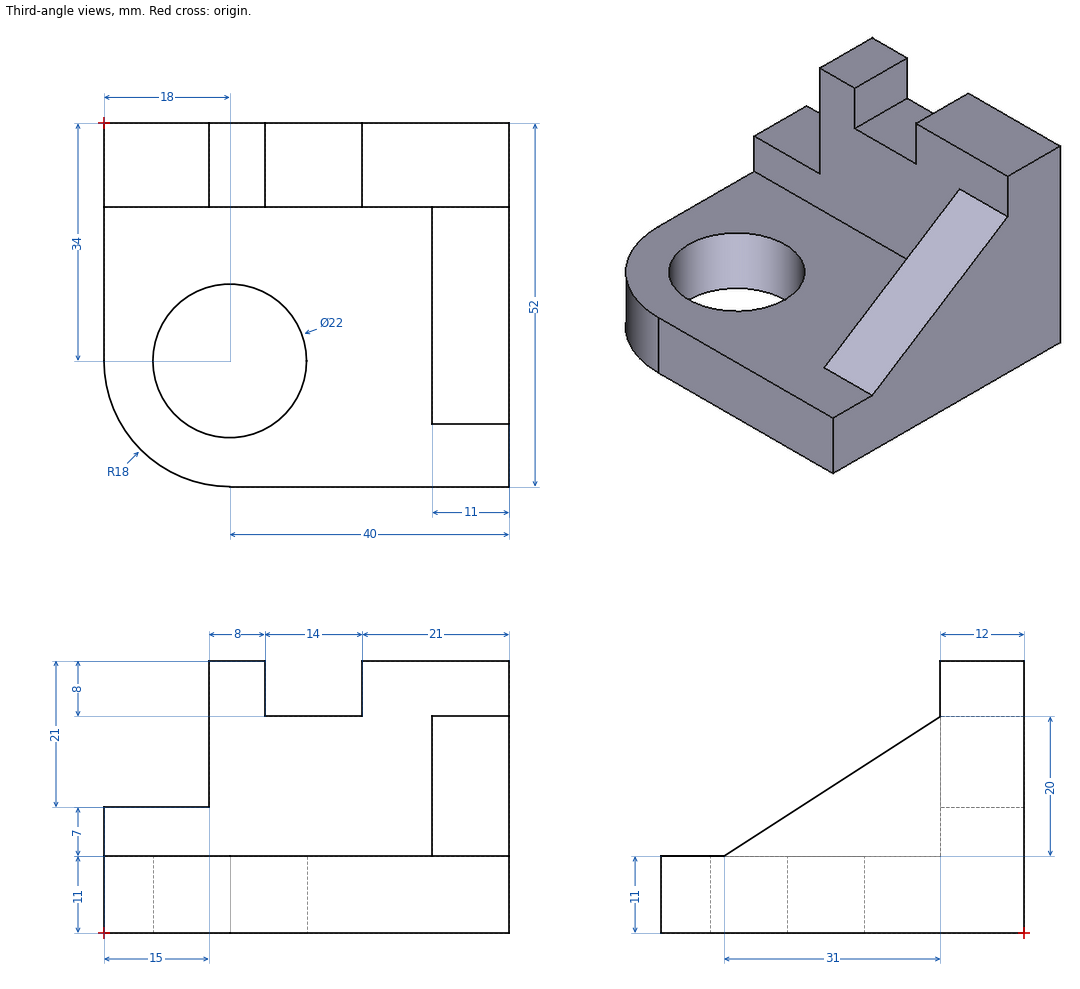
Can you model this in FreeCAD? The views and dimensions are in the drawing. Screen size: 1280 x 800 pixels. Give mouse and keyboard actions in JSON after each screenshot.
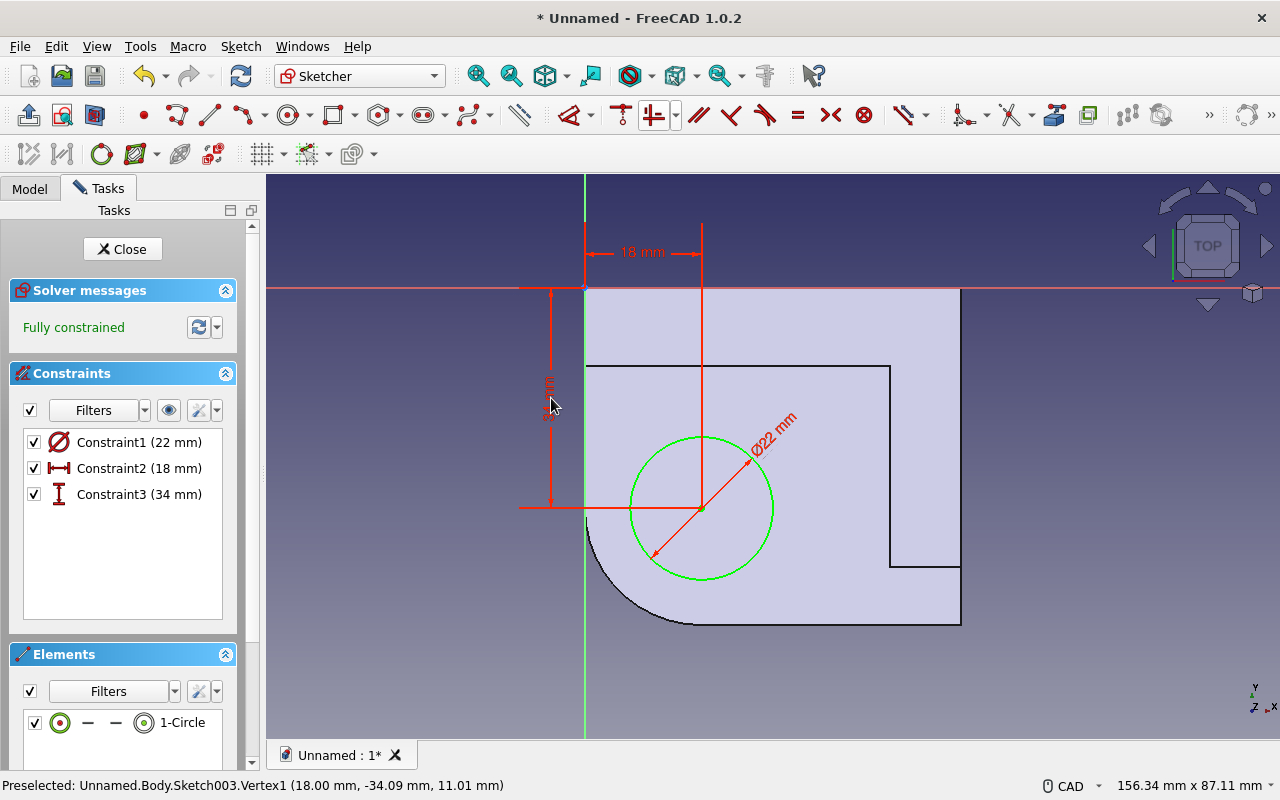
{"action": "left_click", "coordinate": [123, 249]}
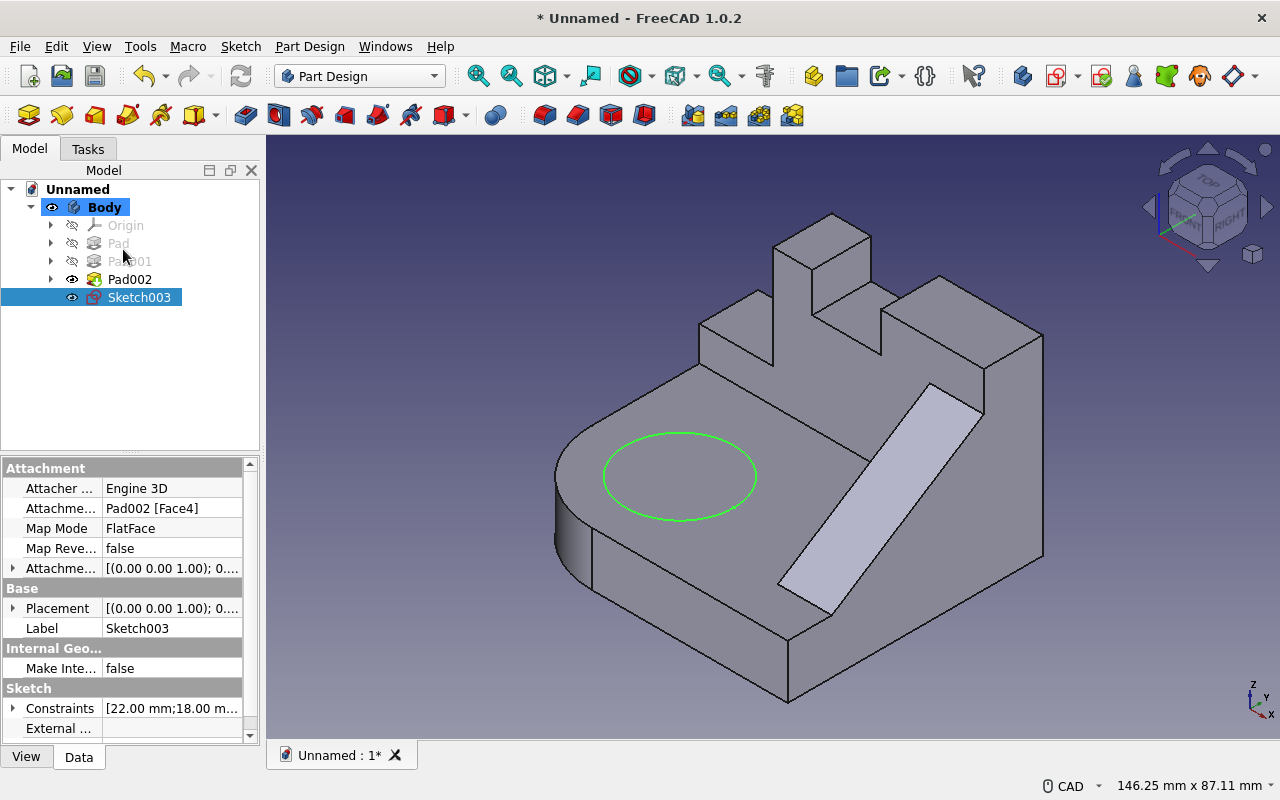
{"action": "left_click", "coordinate": [246, 116]}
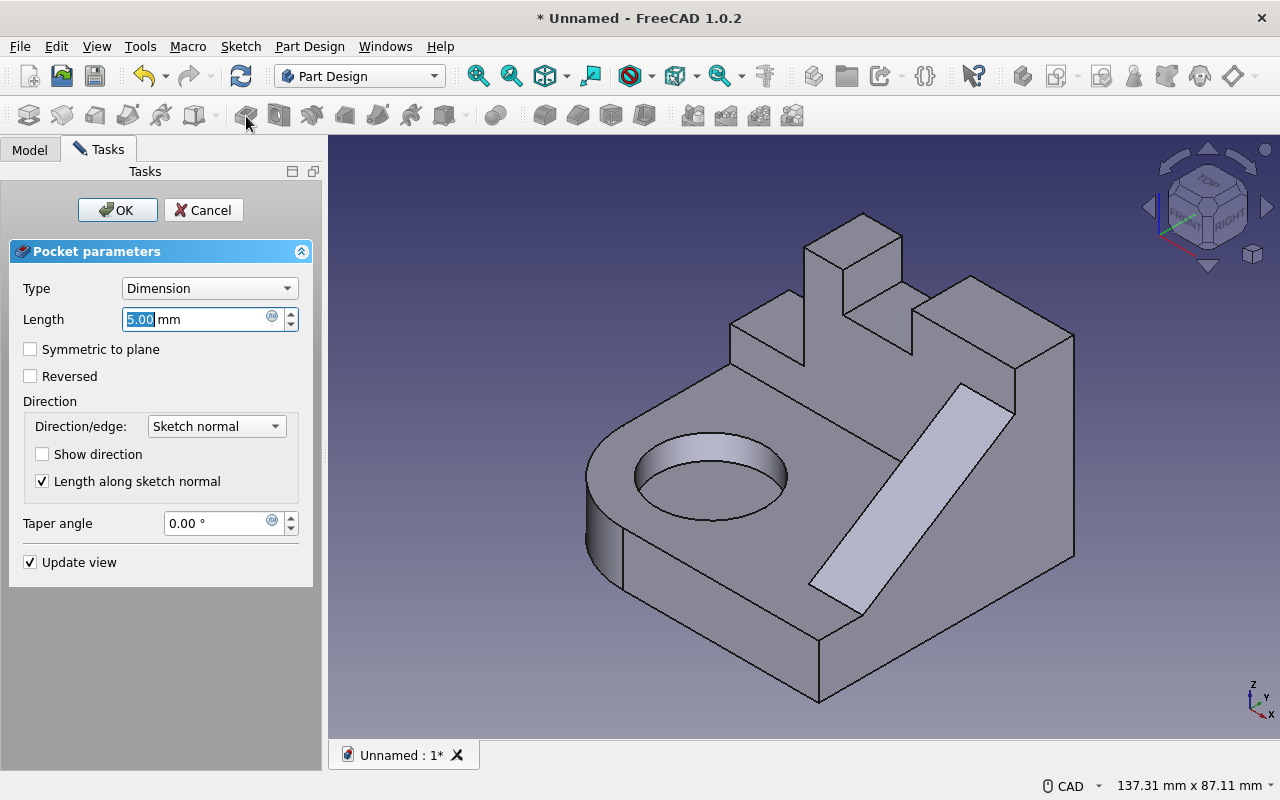
{"action": "type", "text": "11"}
{"action": "key", "text": "Tab"}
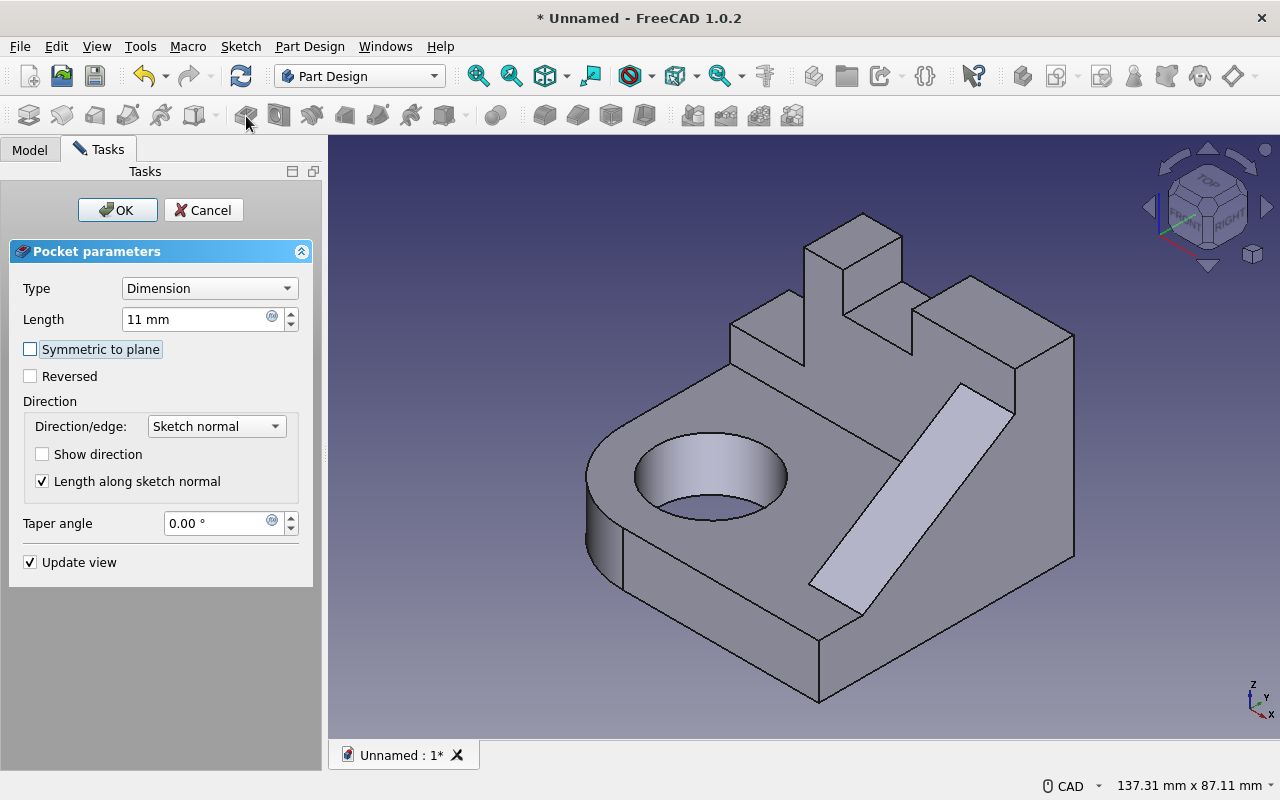
{"action": "left_click", "coordinate": [118, 210]}